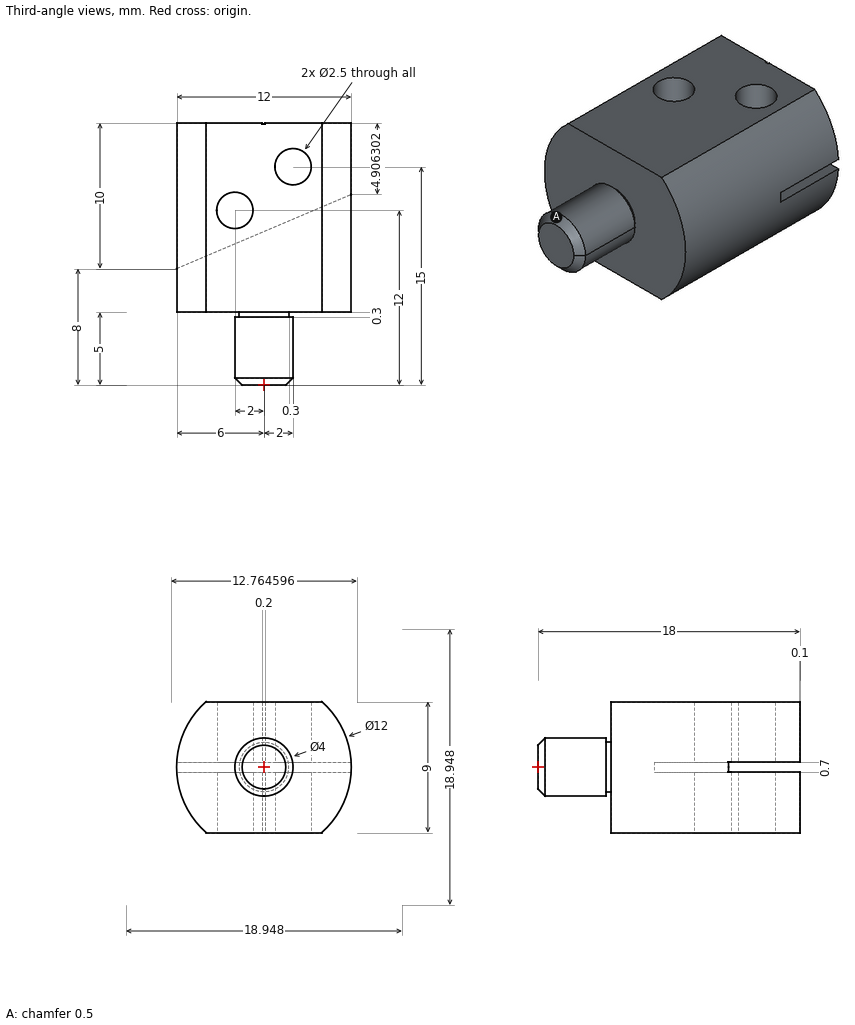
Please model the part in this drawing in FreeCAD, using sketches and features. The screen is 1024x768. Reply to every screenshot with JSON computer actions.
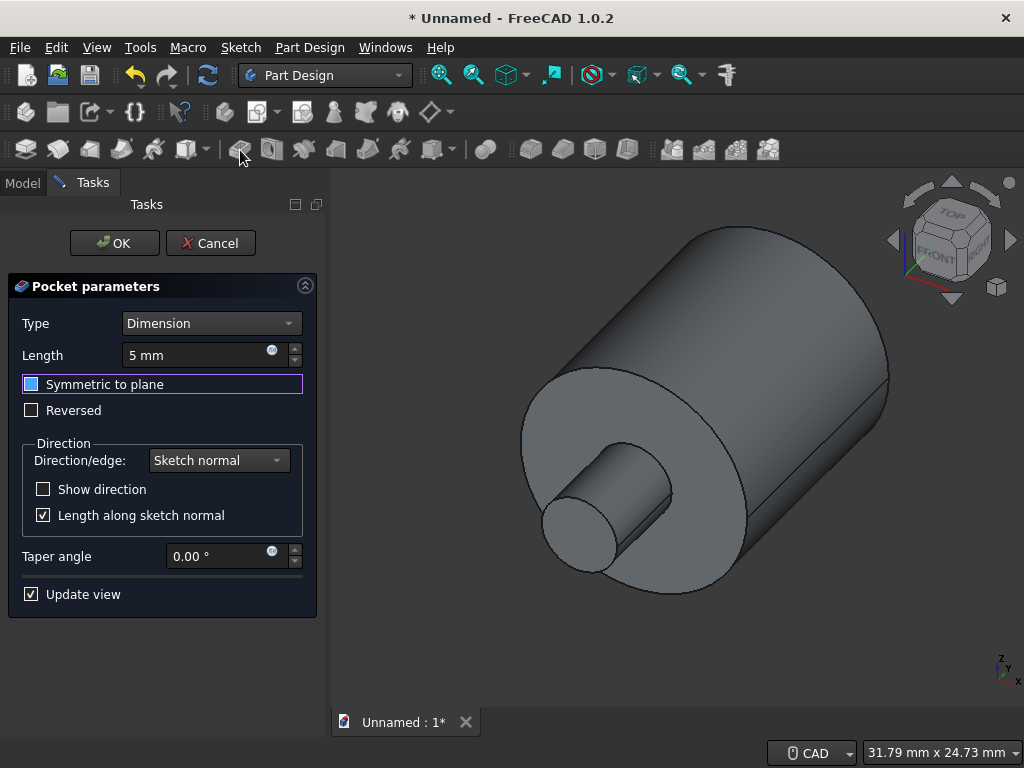
{"action": "left_click", "coordinate": [115, 243]}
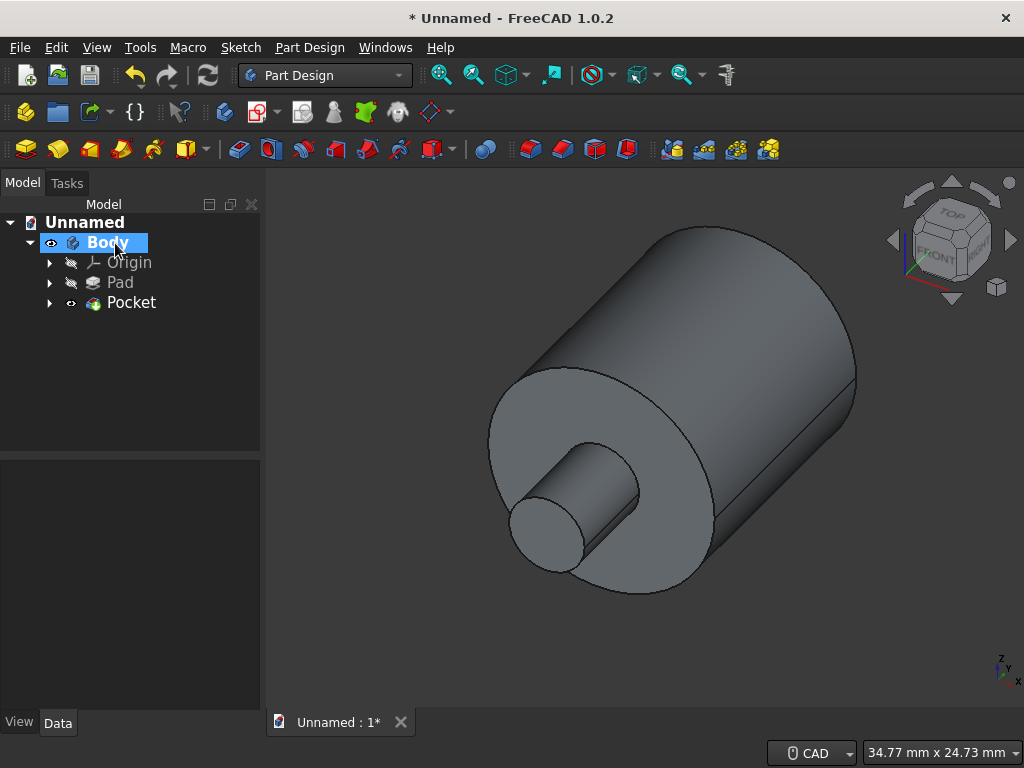
{"action": "left_click", "coordinate": [258, 112]}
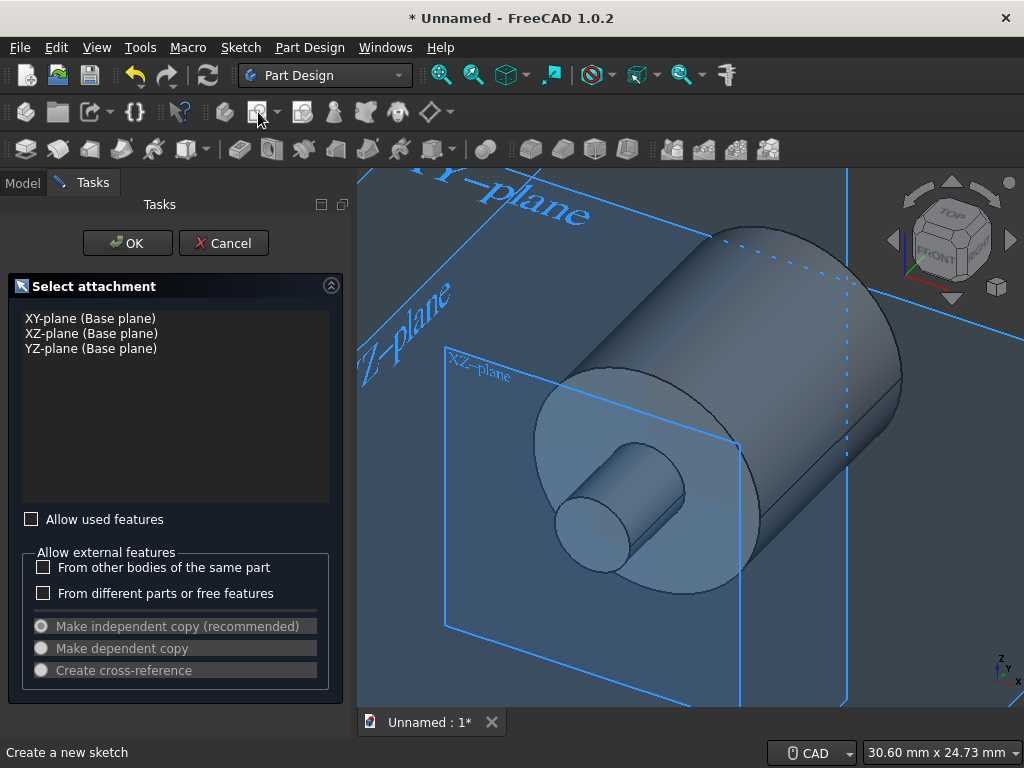
{"action": "left_click", "coordinate": [82, 318]}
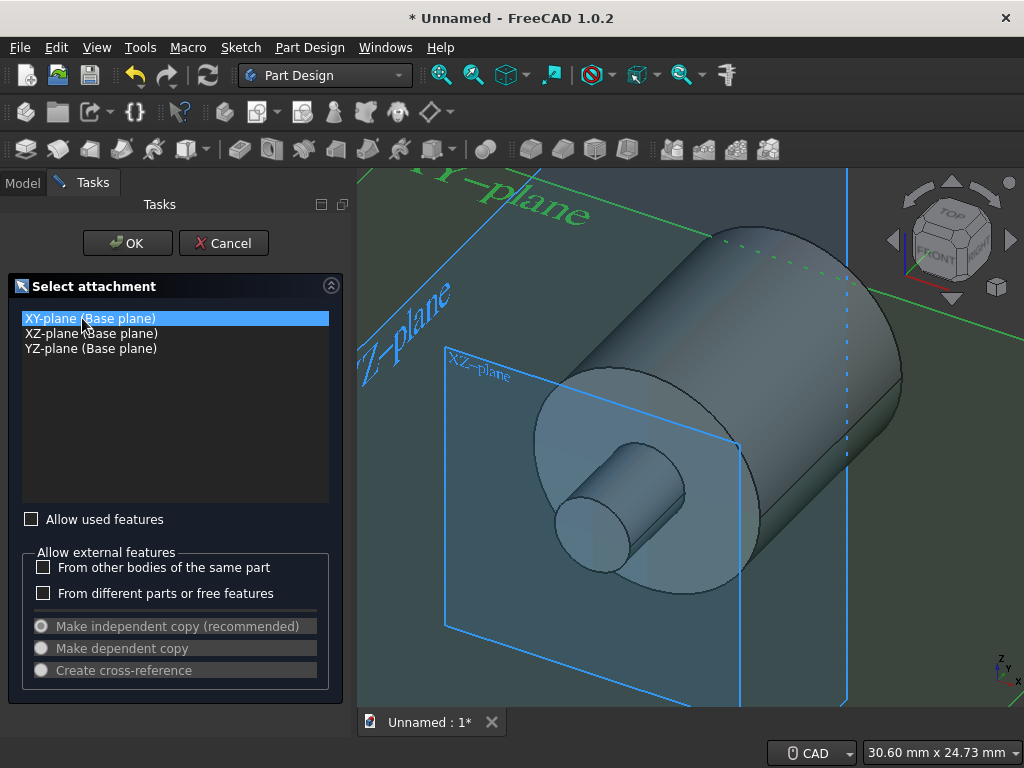
{"action": "left_click", "coordinate": [128, 243]}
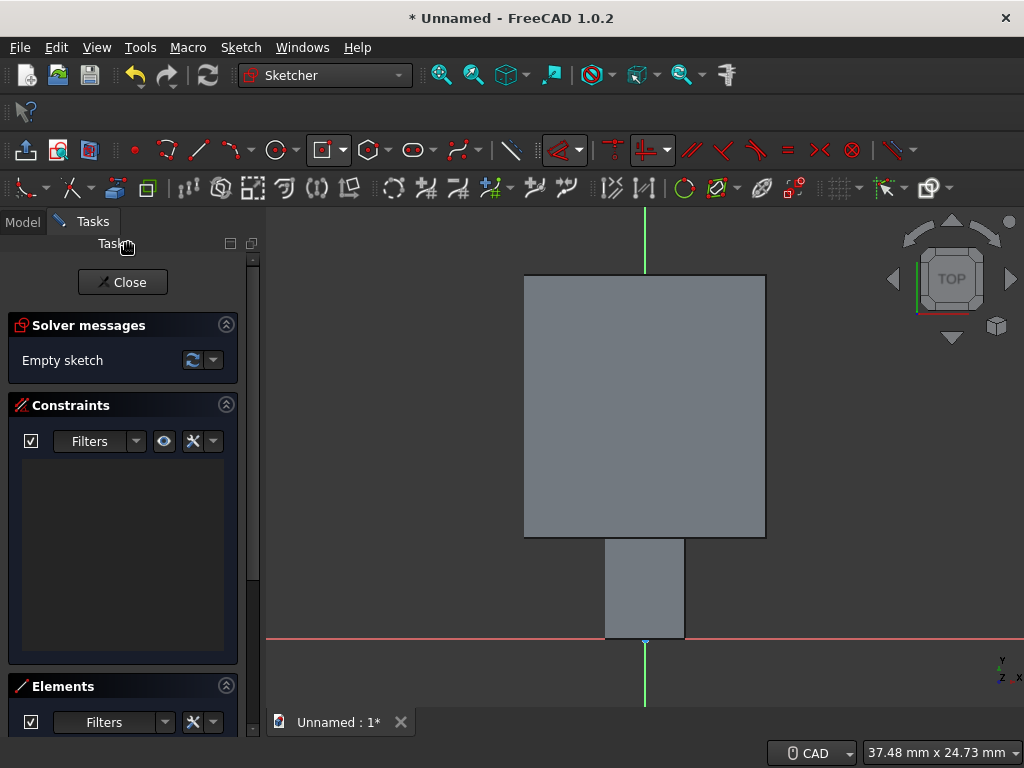
{"action": "left_click", "coordinate": [90, 150]}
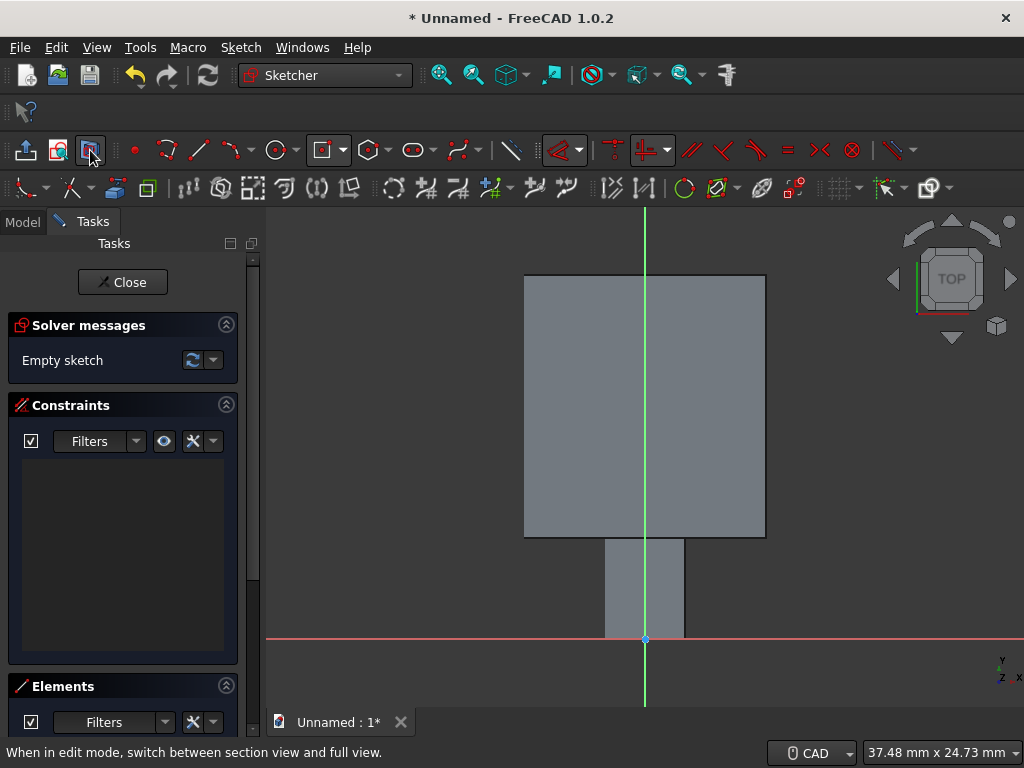
{"action": "key", "text": "g m"}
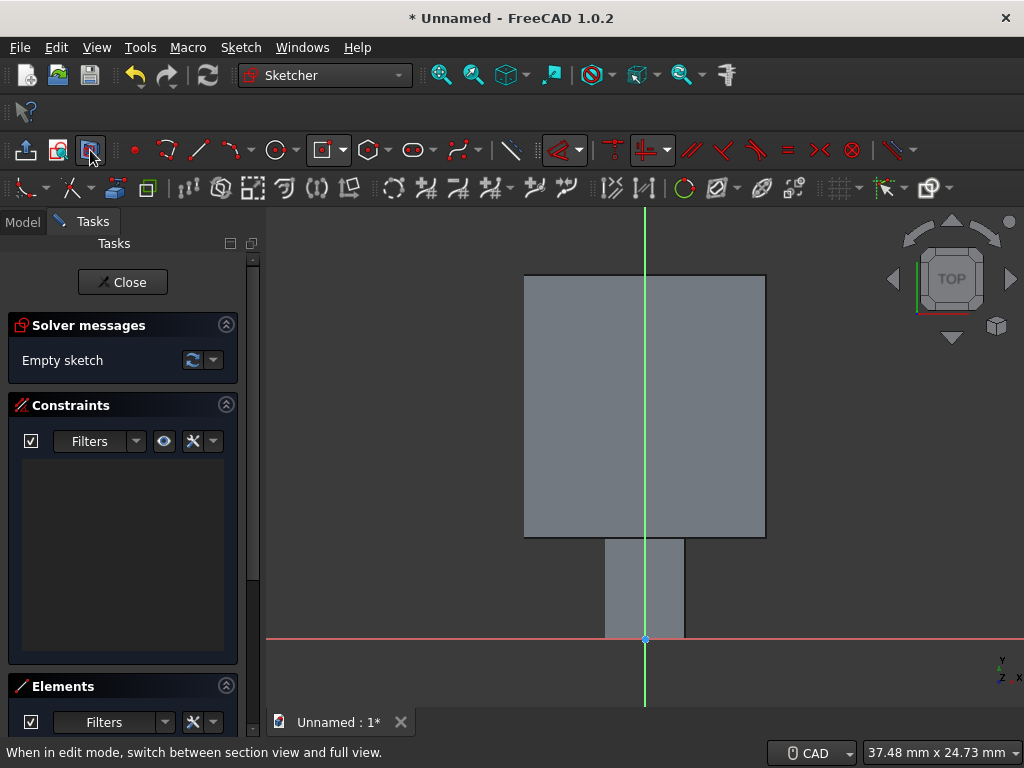
{"action": "left_click", "coordinate": [524, 477]}
{"action": "left_click", "coordinate": [766, 374]}
{"action": "left_click", "coordinate": [766, 275]}
{"action": "left_click", "coordinate": [524, 275]}
{"action": "left_click", "coordinate": [524, 478]}
{"action": "key", "text": "Escape"}
{"action": "key", "text": "Escape"}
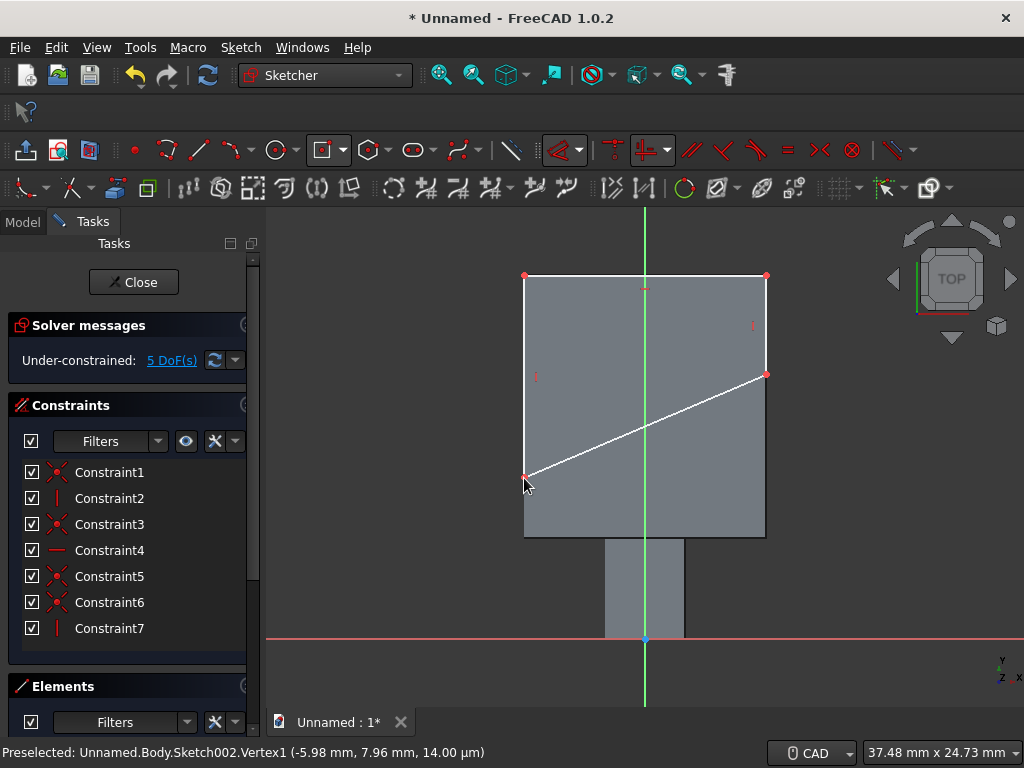
{"action": "left_click", "coordinate": [693, 276]}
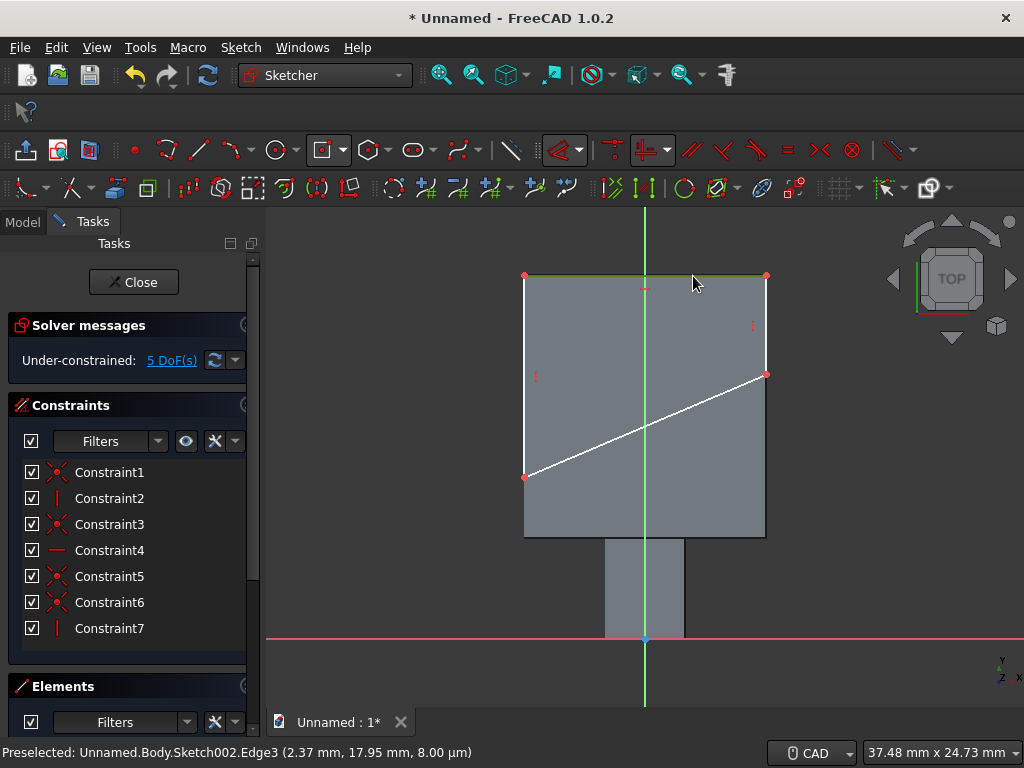
{"action": "left_click", "coordinate": [582, 150]}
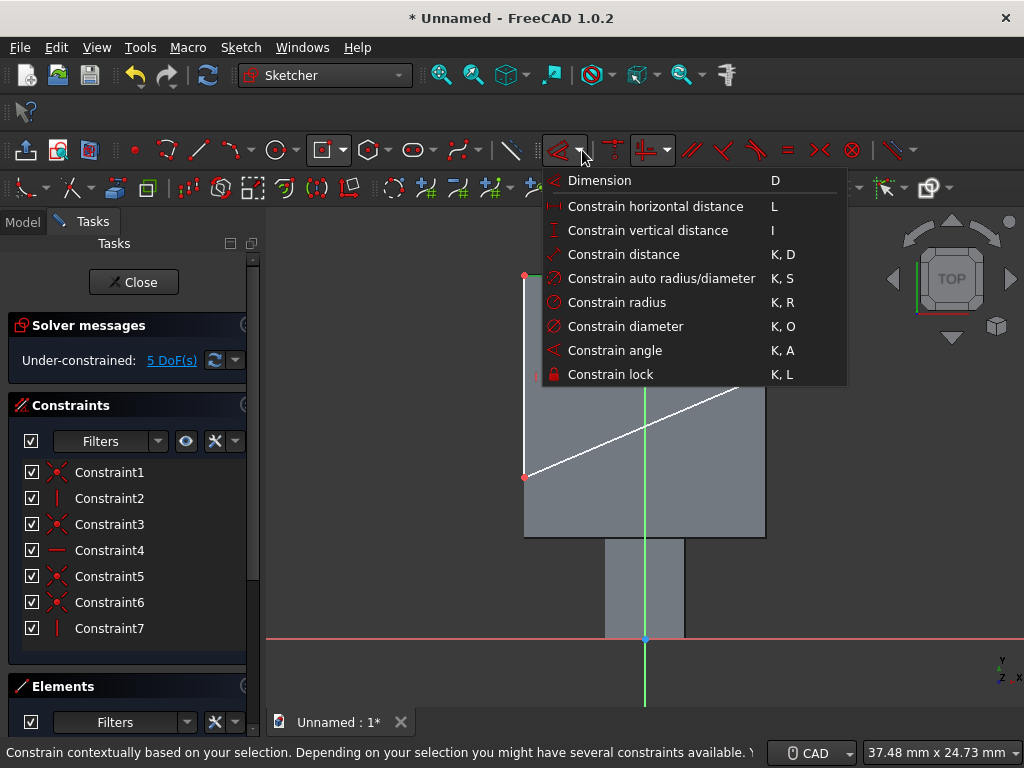
{"action": "left_click", "coordinate": [695, 206]}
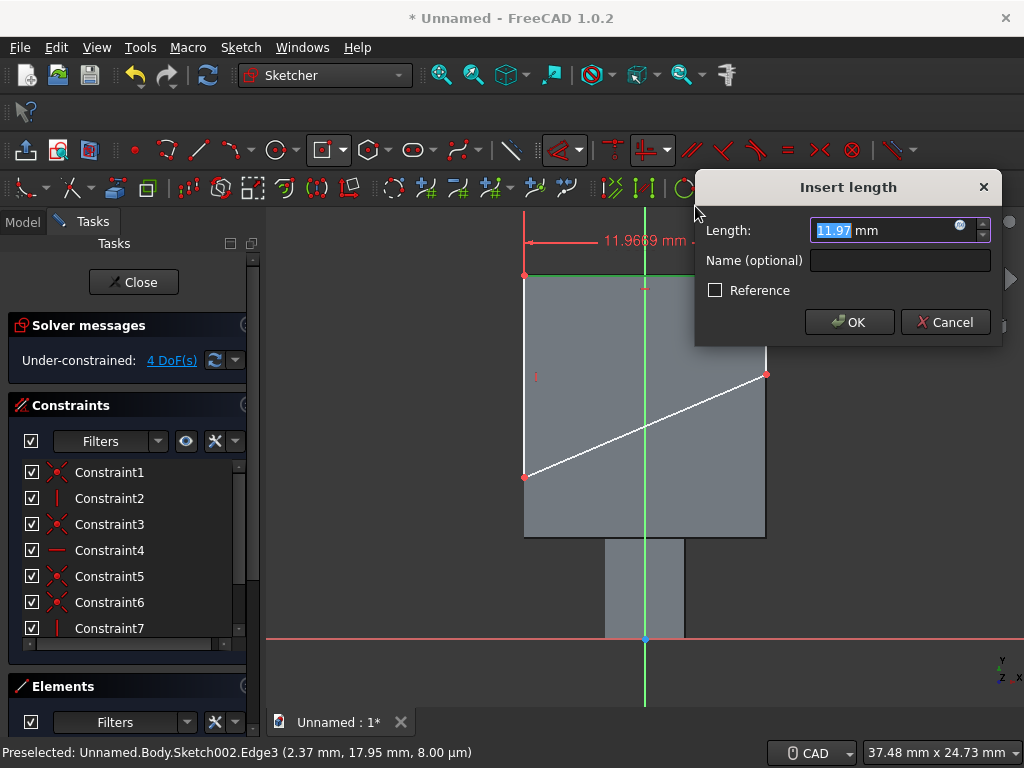
{"action": "type", "text": "12"}
{"action": "key", "text": "Return"}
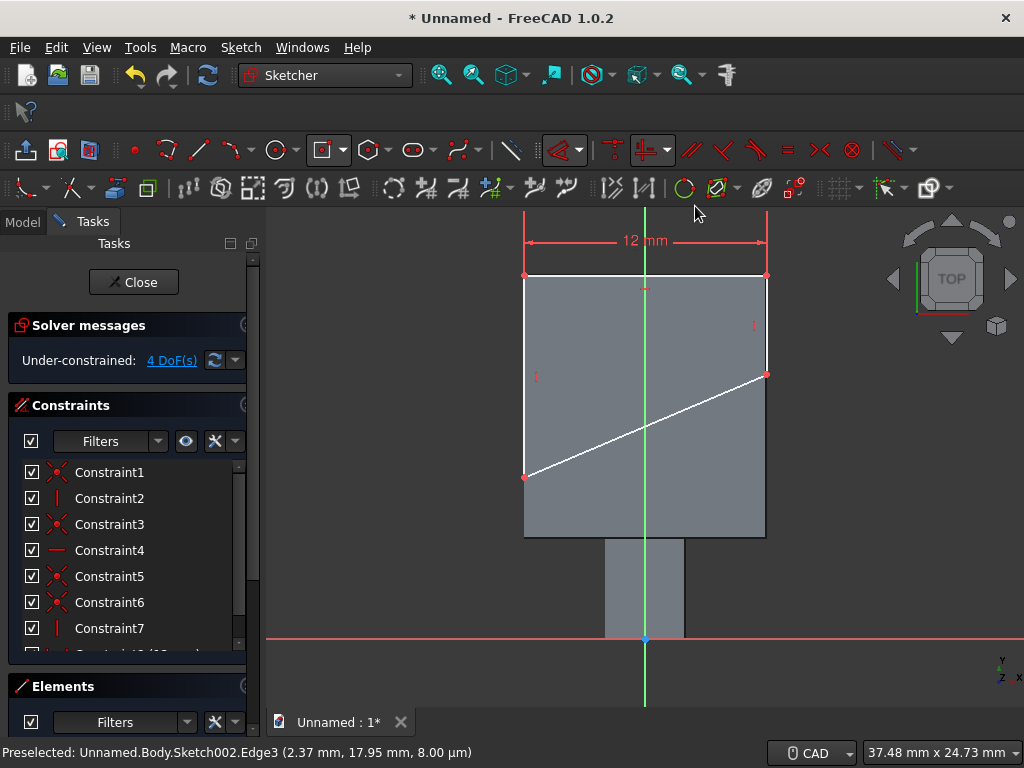
{"action": "left_click", "coordinate": [524, 337]}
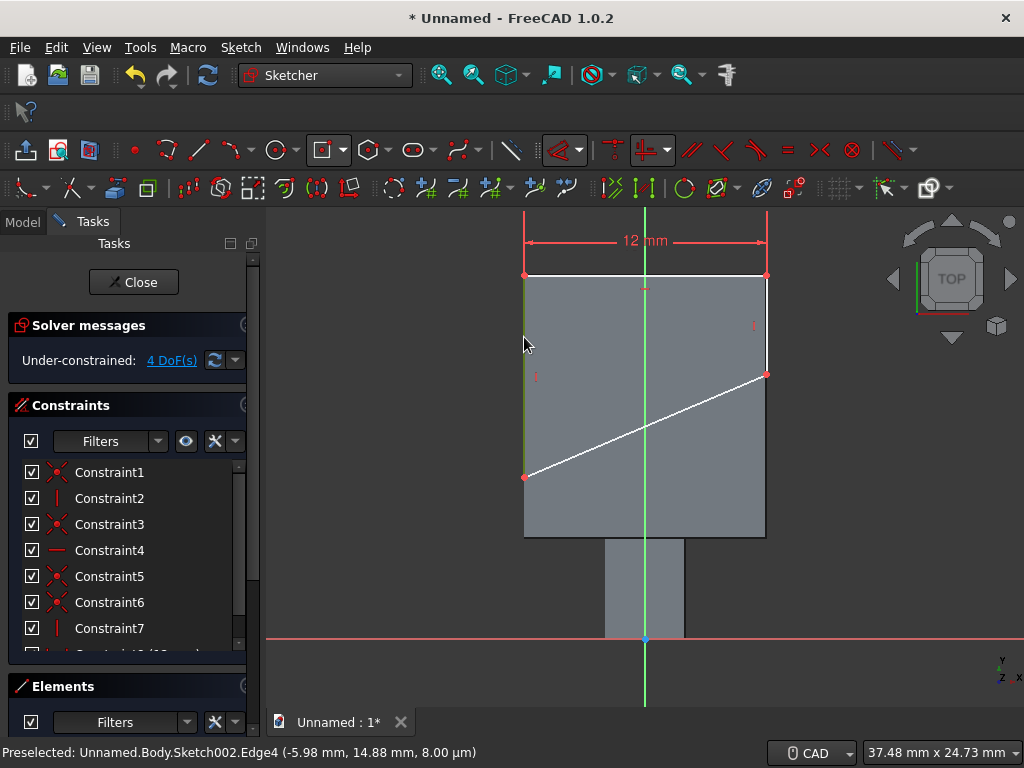
{"action": "left_click", "coordinate": [582, 150]}